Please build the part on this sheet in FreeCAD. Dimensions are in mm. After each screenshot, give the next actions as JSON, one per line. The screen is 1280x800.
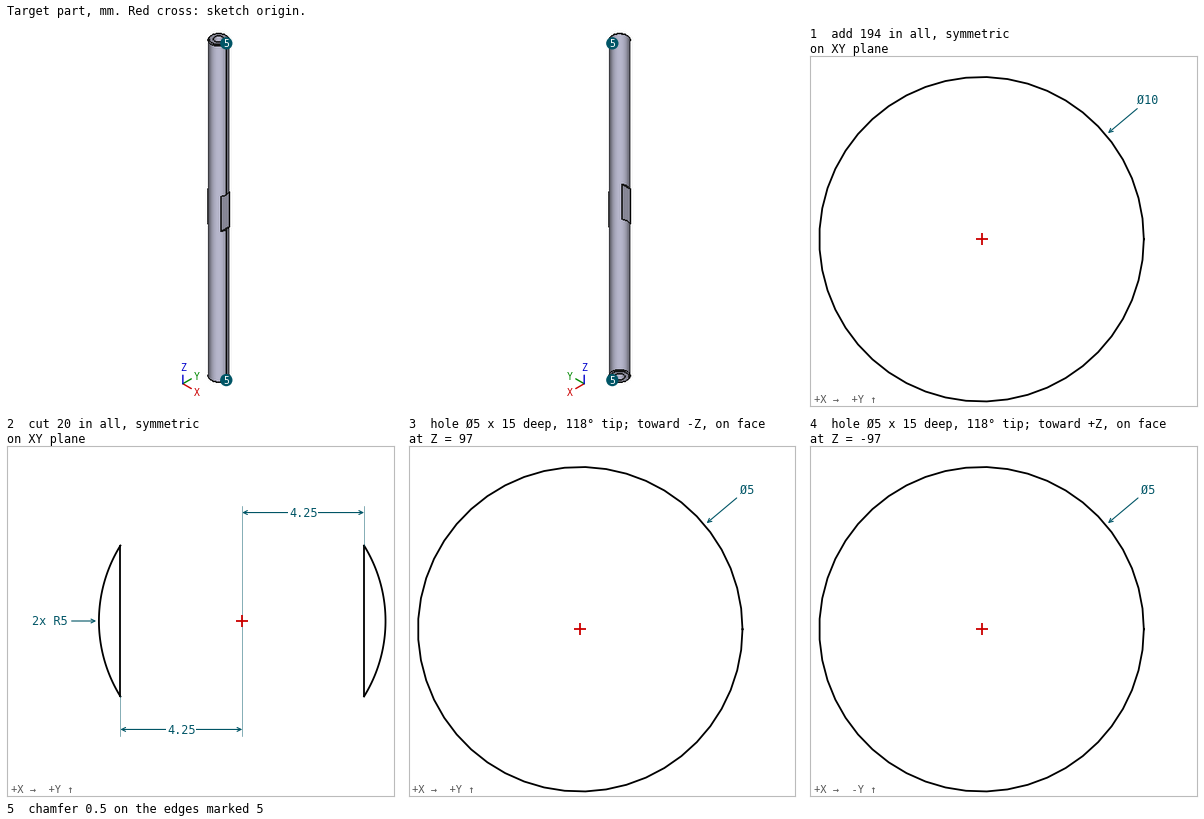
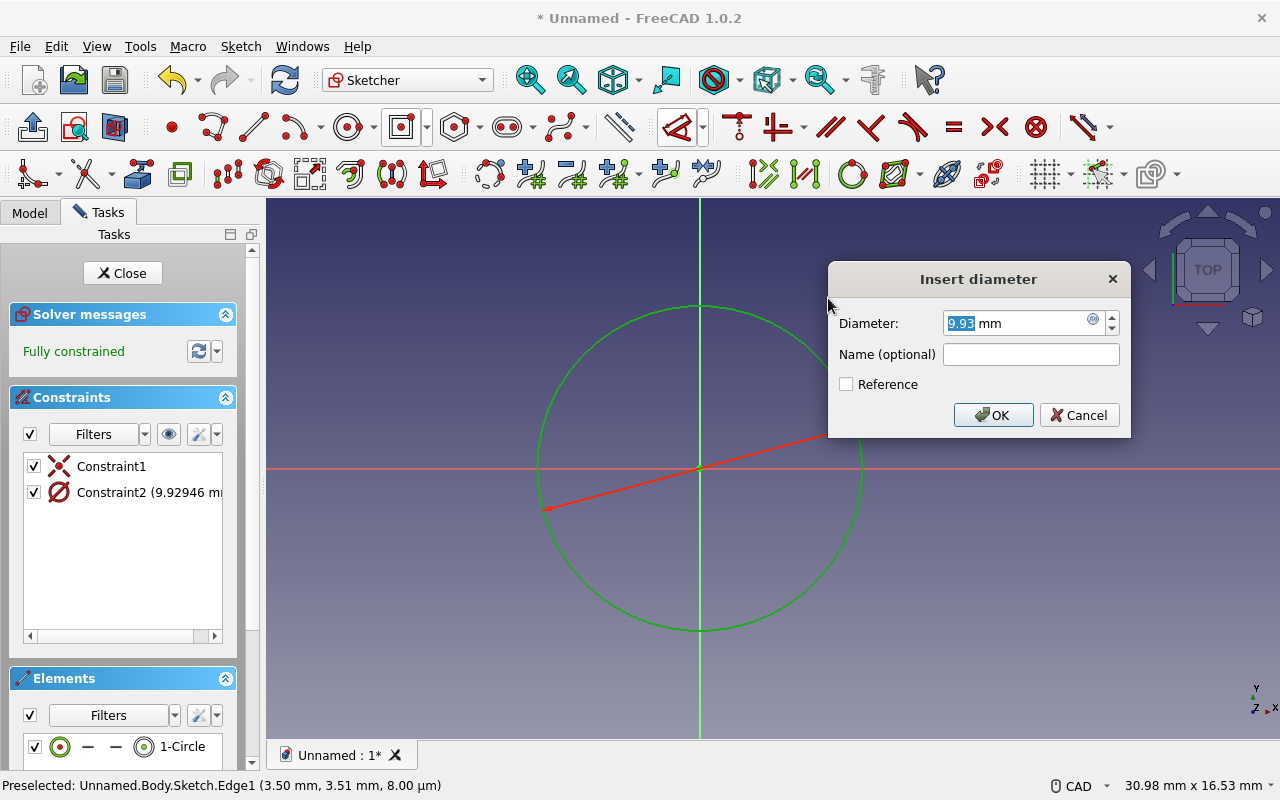
{"action": "type", "text": "10"}
{"action": "key", "text": "Return"}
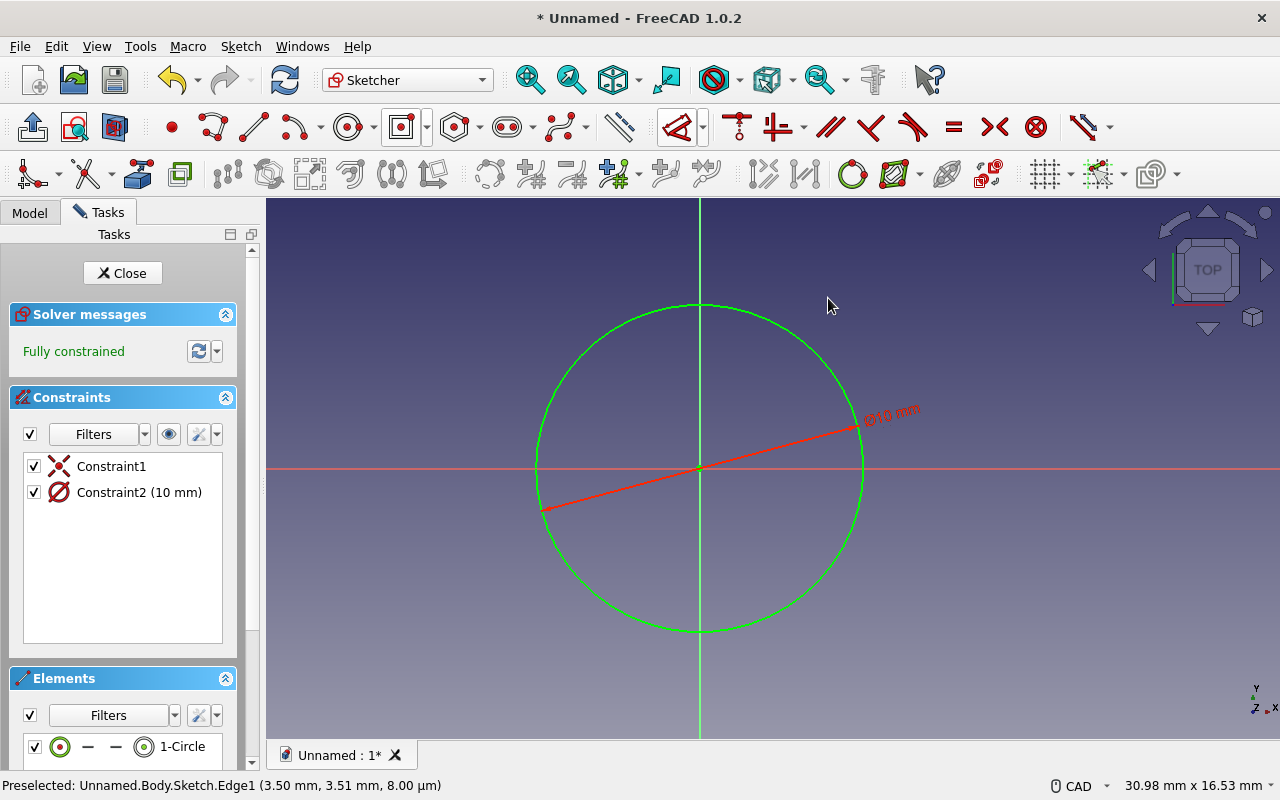
{"action": "left_click", "coordinate": [123, 273]}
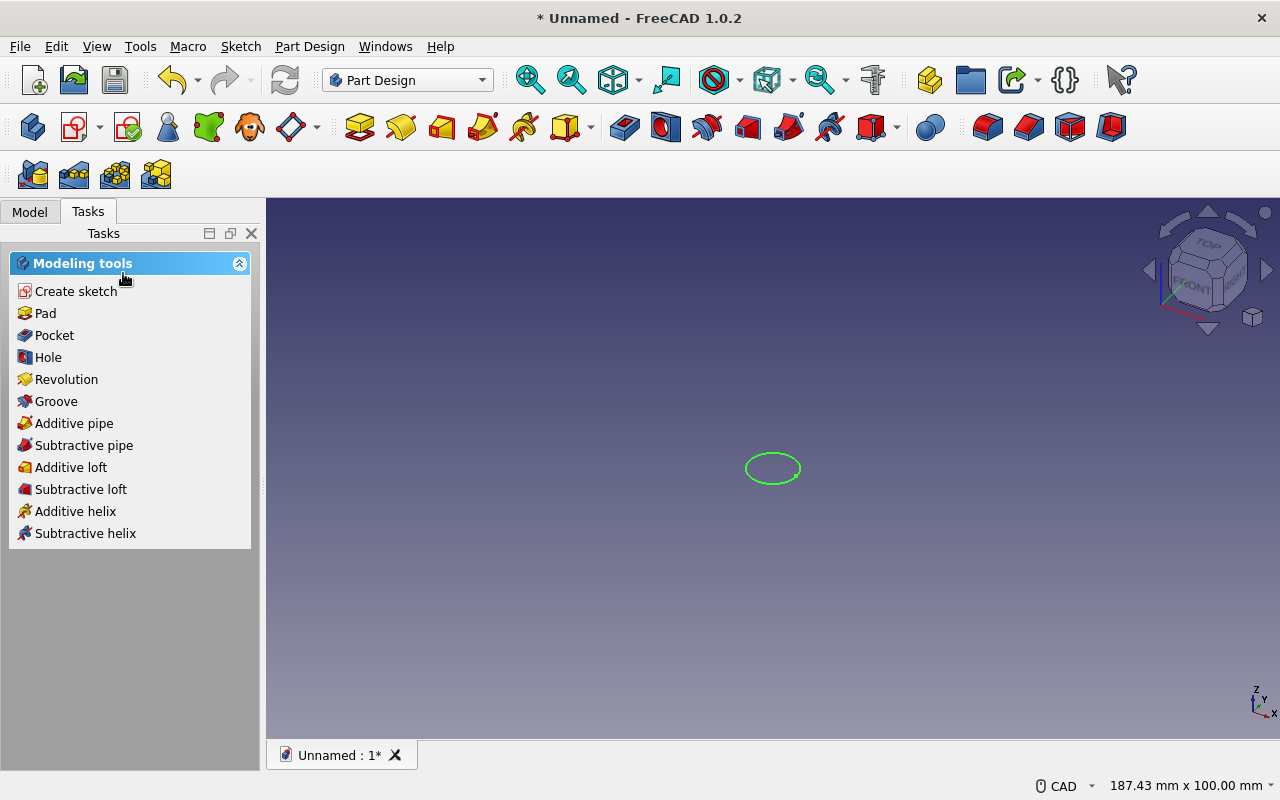
{"action": "left_click", "coordinate": [360, 128]}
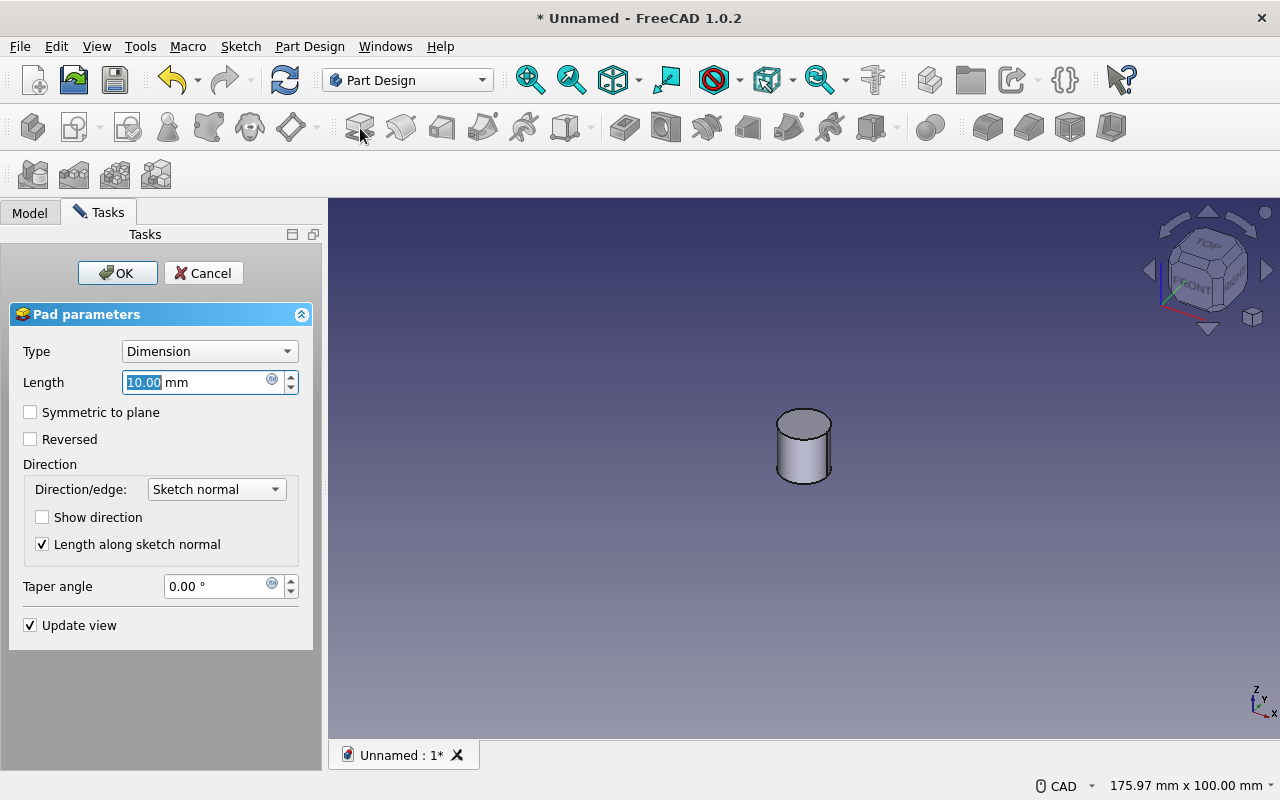
{"action": "type", "text": "194"}
{"action": "key", "text": "Tab"}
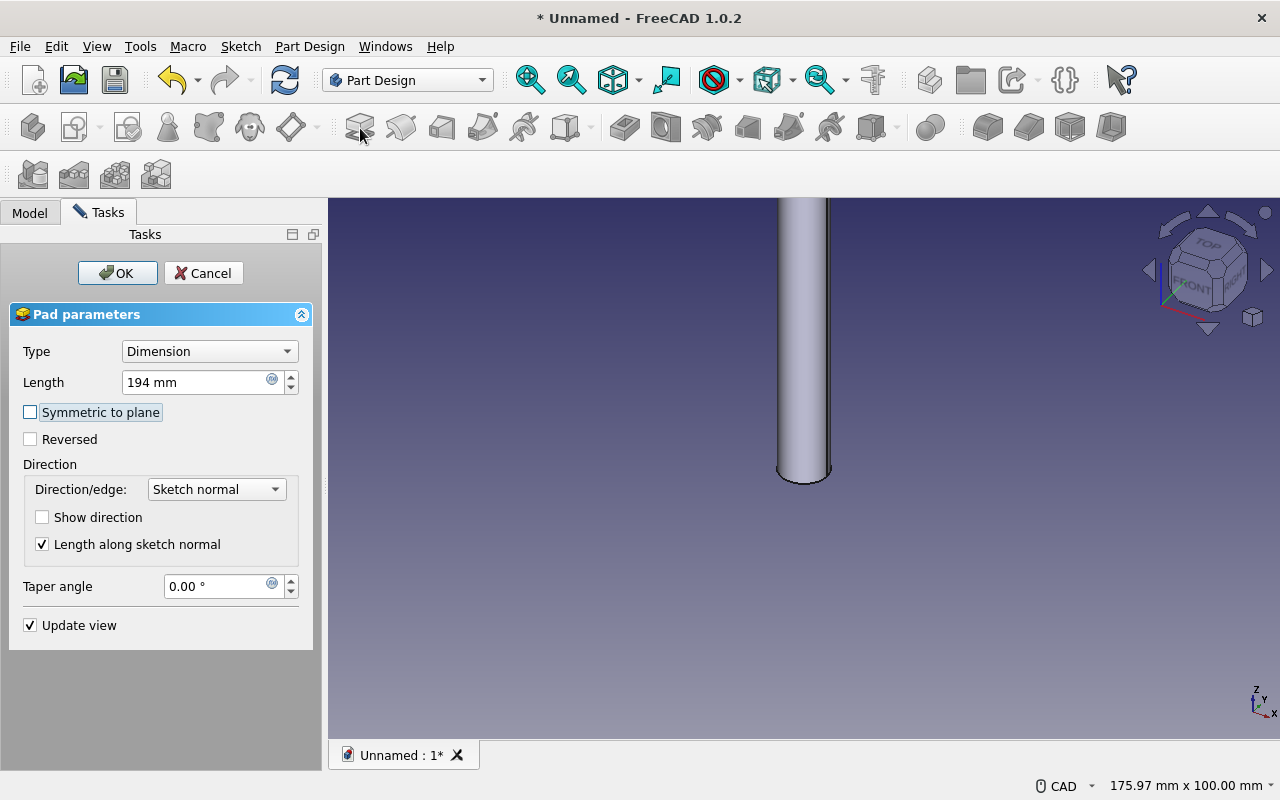
{"action": "left_click", "coordinate": [31, 412]}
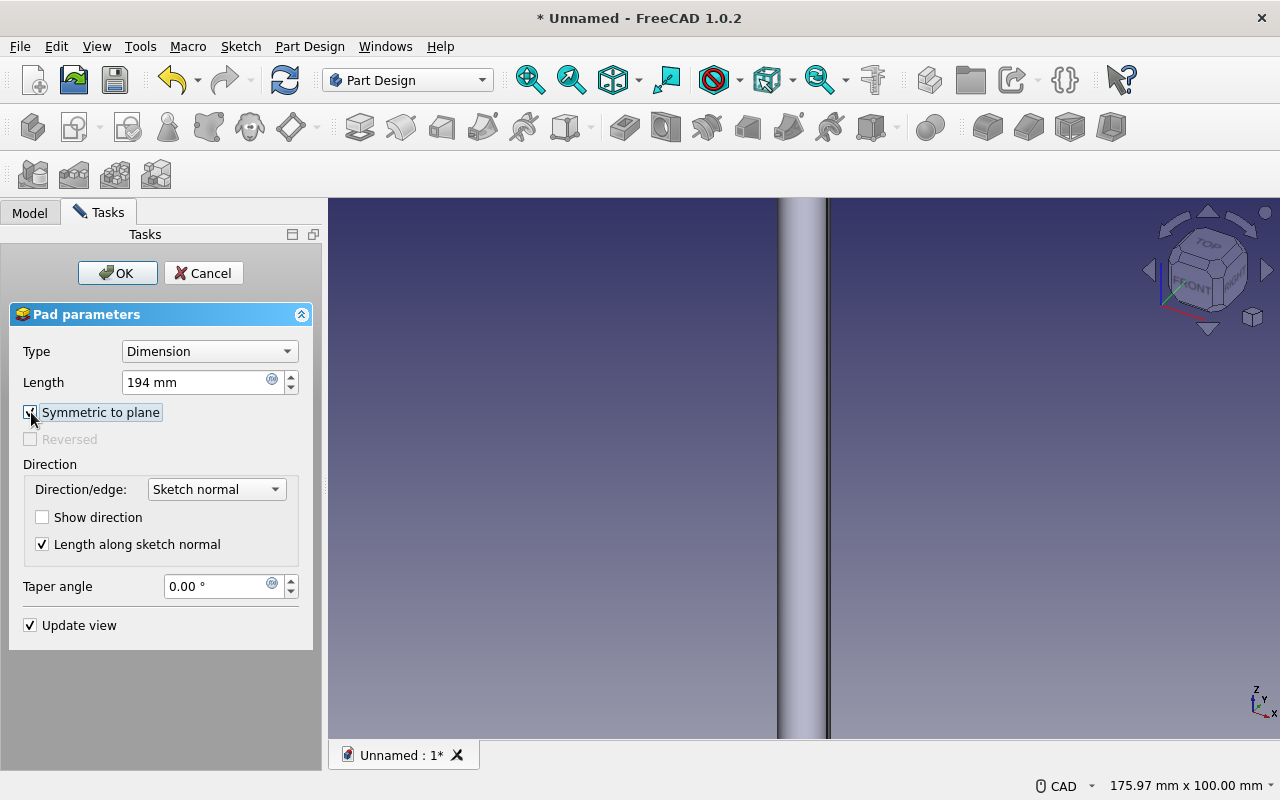
{"action": "left_click", "coordinate": [118, 273]}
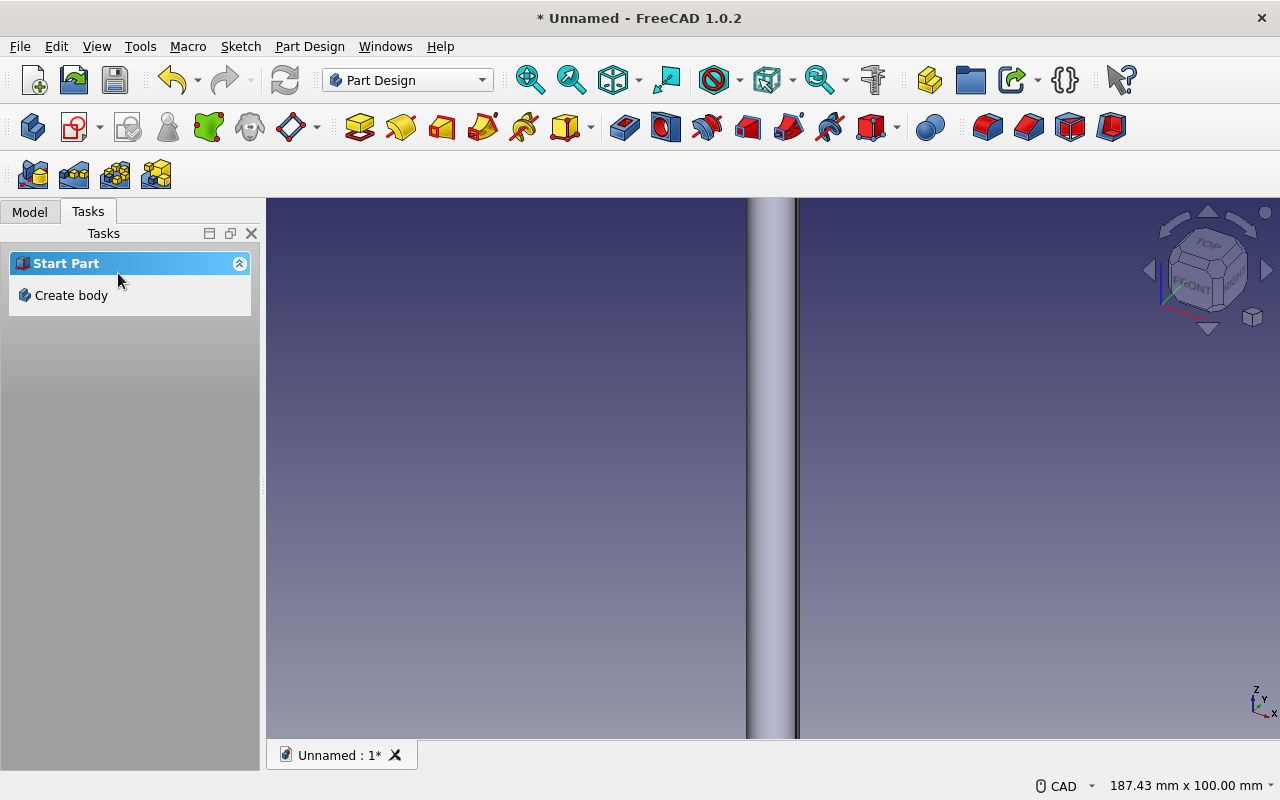
{"action": "left_click", "coordinate": [531, 80]}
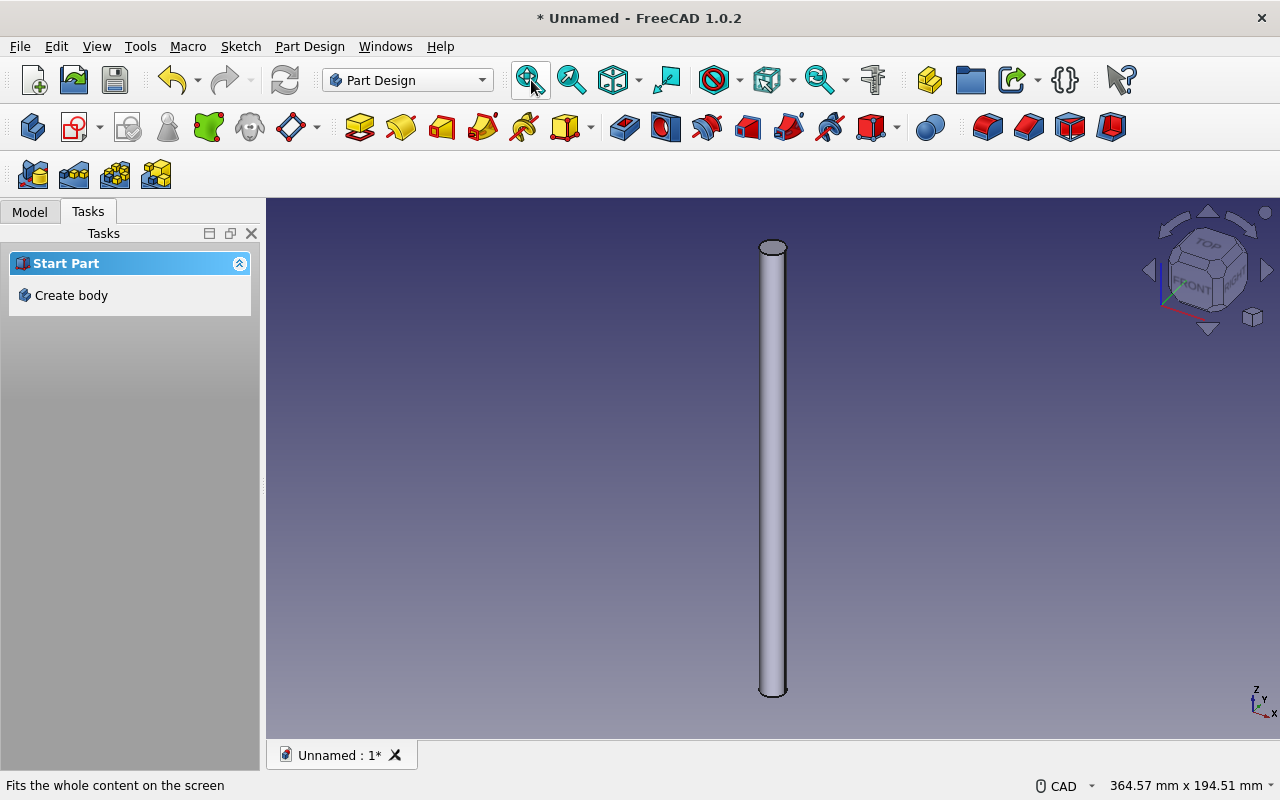
{"action": "left_click", "coordinate": [74, 128]}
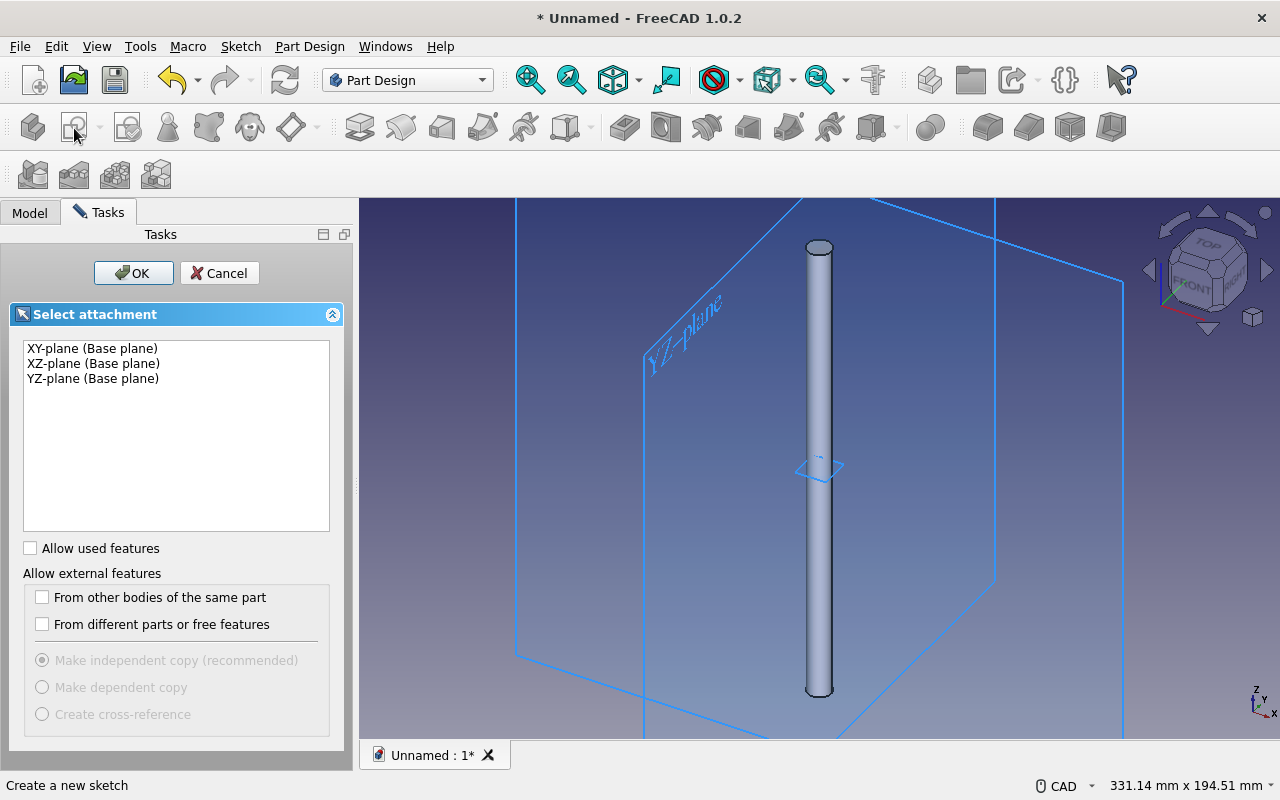
{"action": "left_click", "coordinate": [84, 348]}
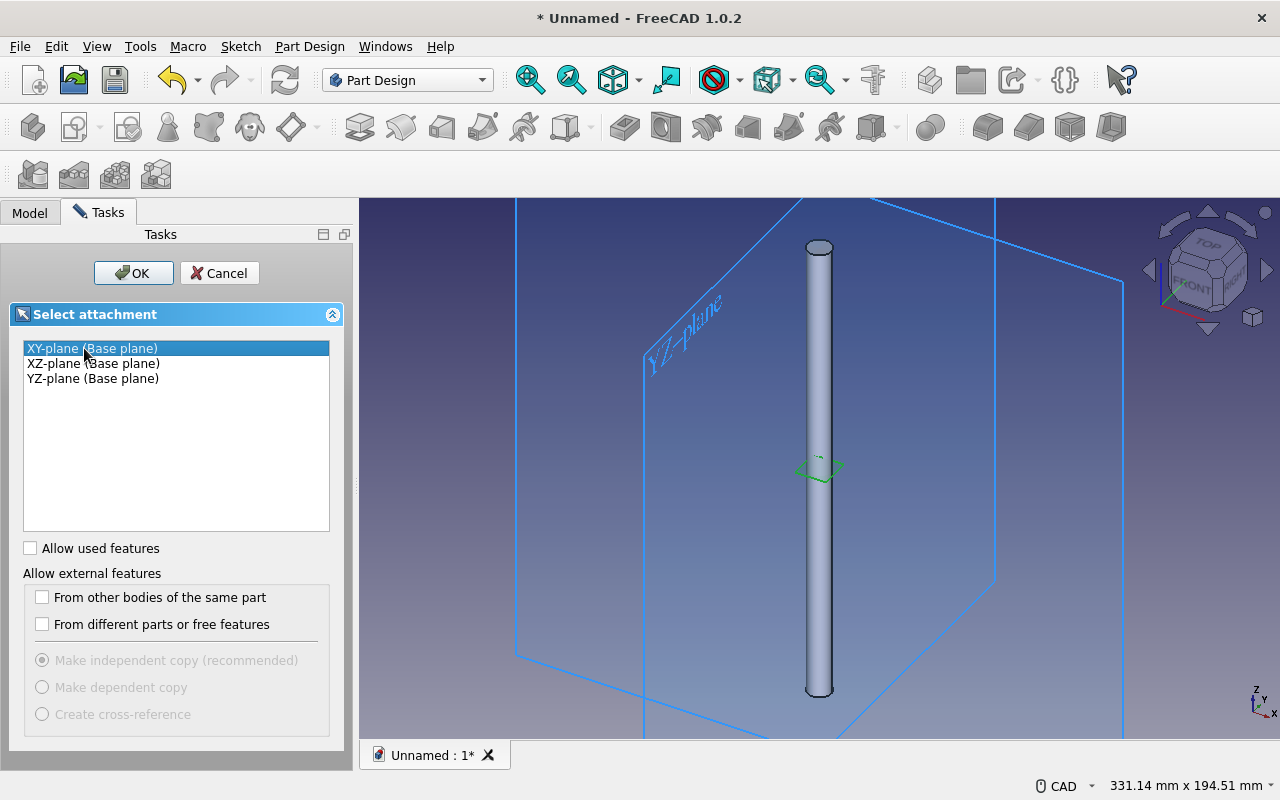
{"action": "left_click", "coordinate": [134, 273]}